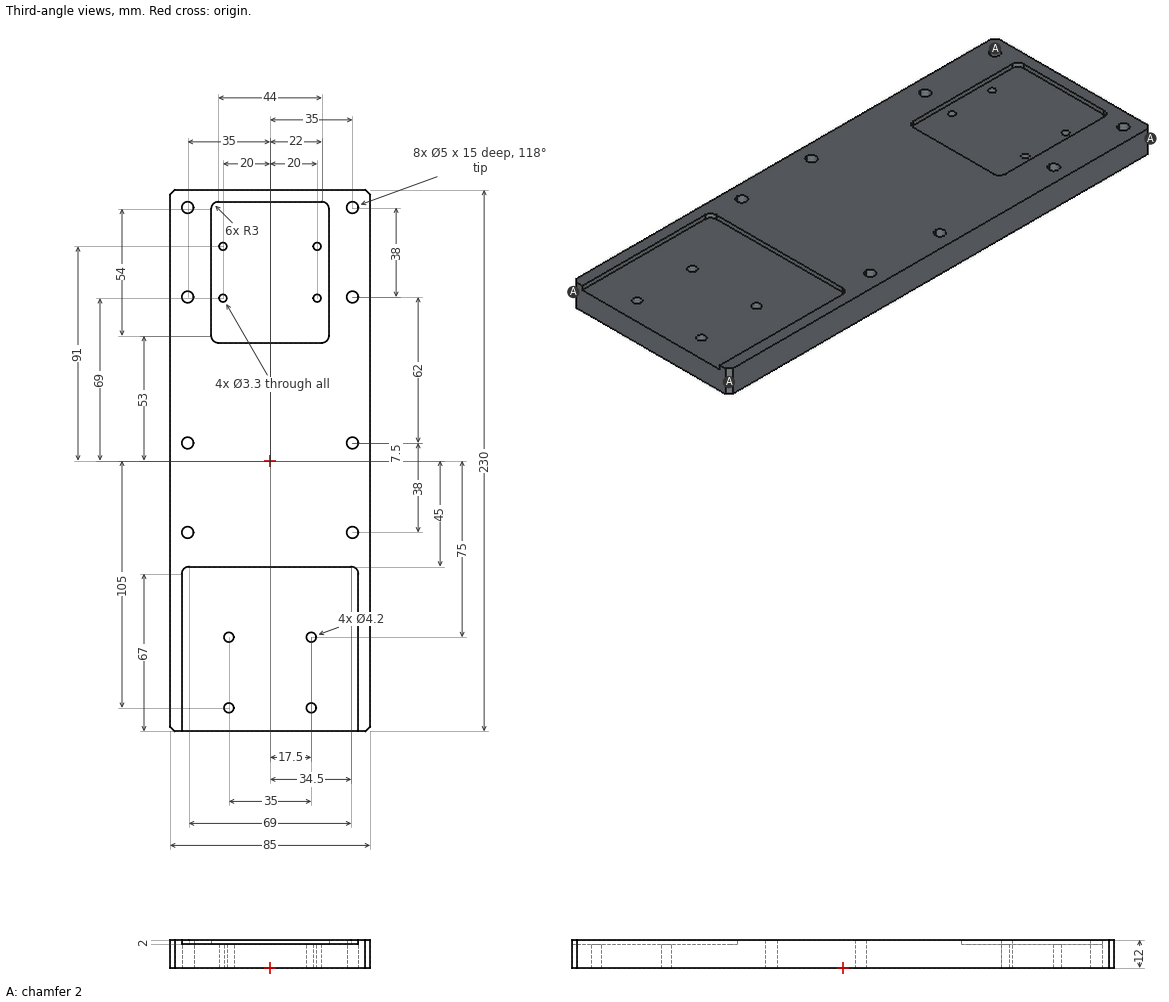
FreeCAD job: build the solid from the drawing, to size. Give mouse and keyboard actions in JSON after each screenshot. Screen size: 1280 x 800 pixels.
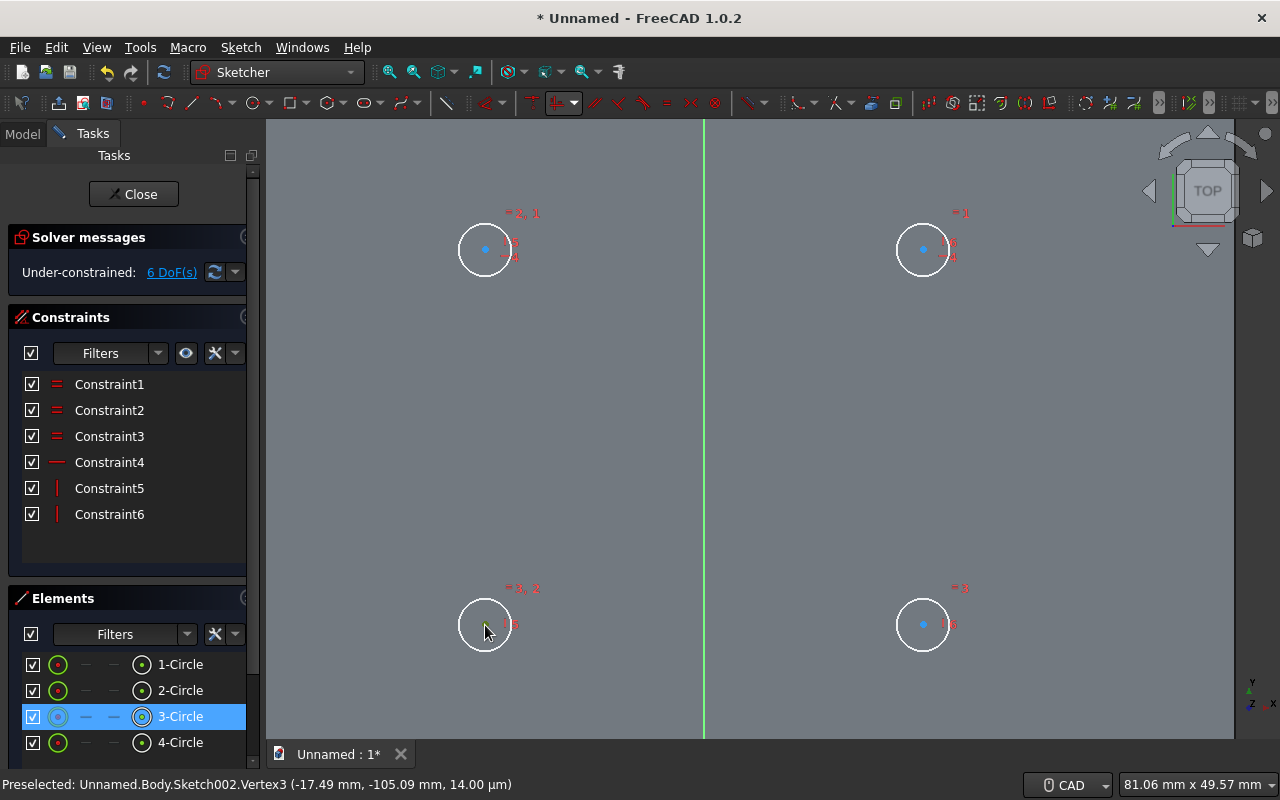
{"action": "left_click", "coordinate": [923, 625]}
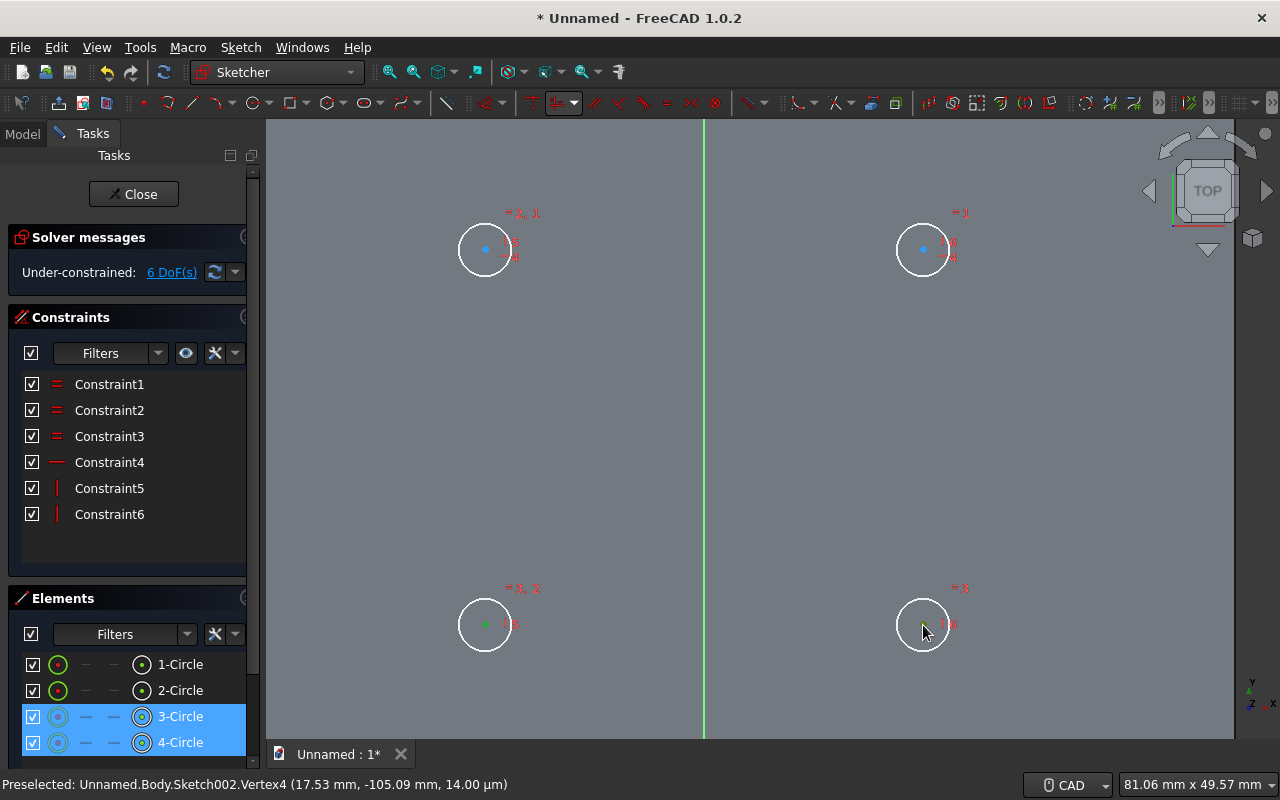
{"action": "key", "text": "h"}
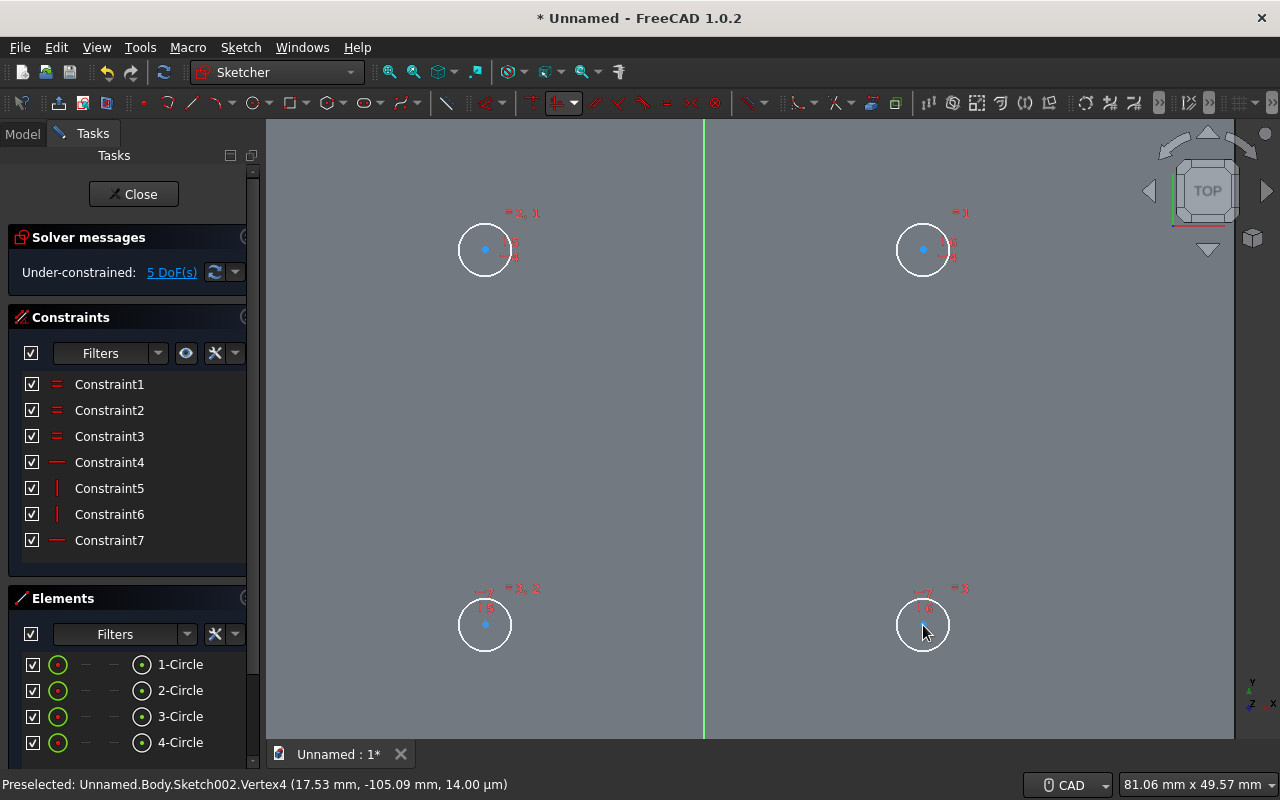
{"action": "left_click", "coordinate": [941, 231]}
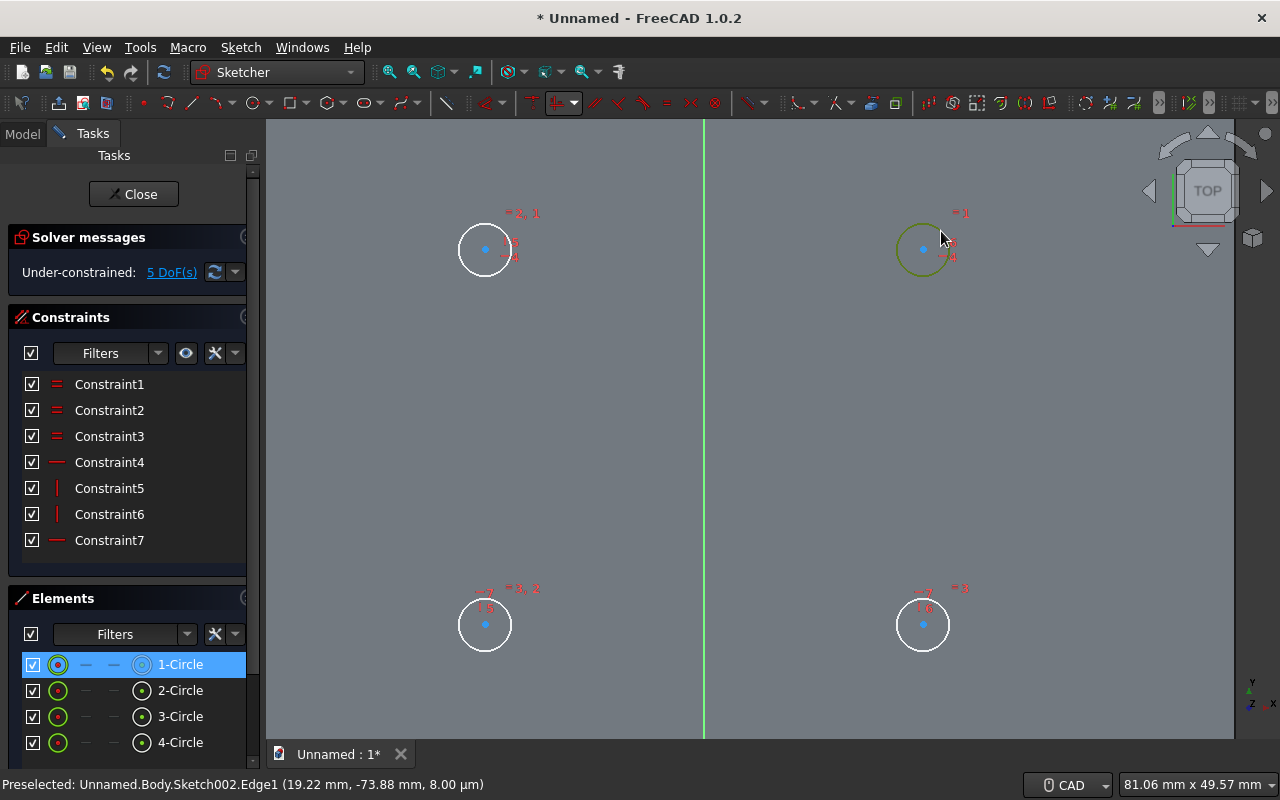
{"action": "left_click", "coordinate": [504, 104]}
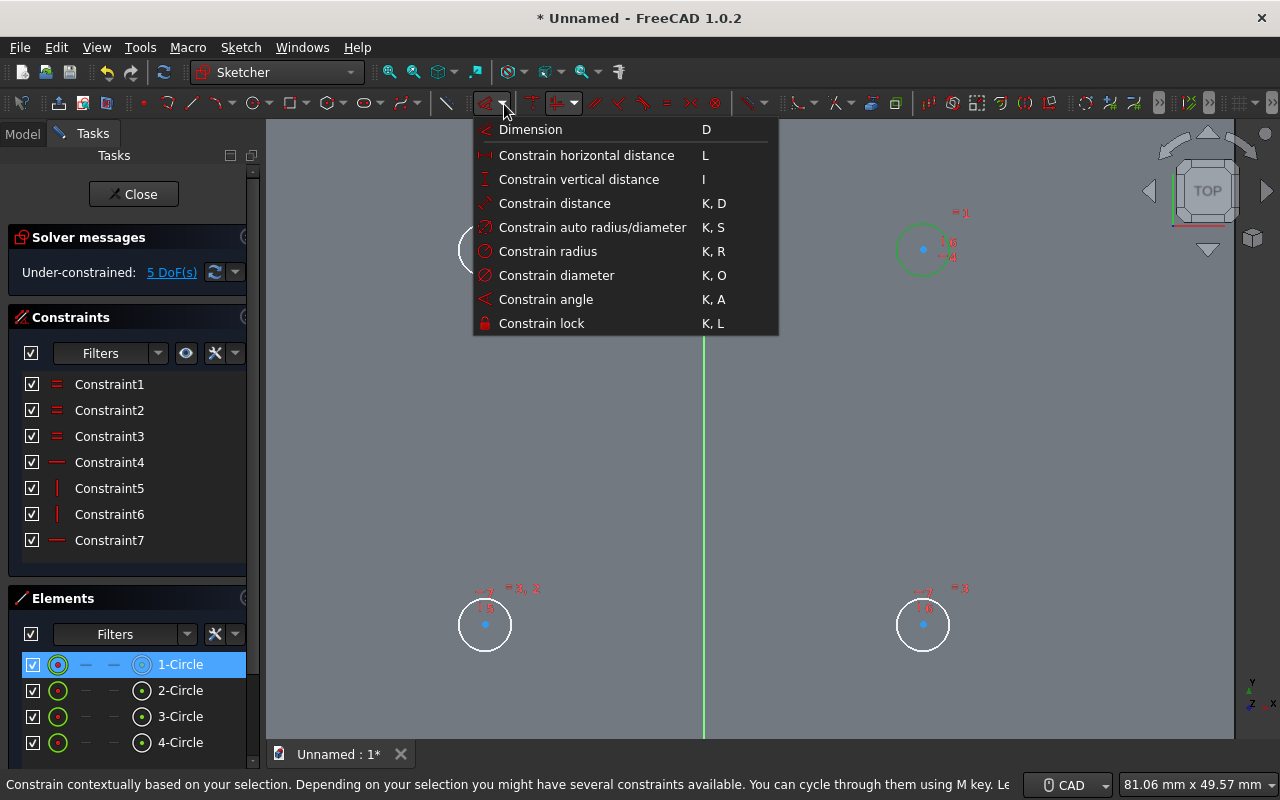
{"action": "left_click", "coordinate": [626, 275]}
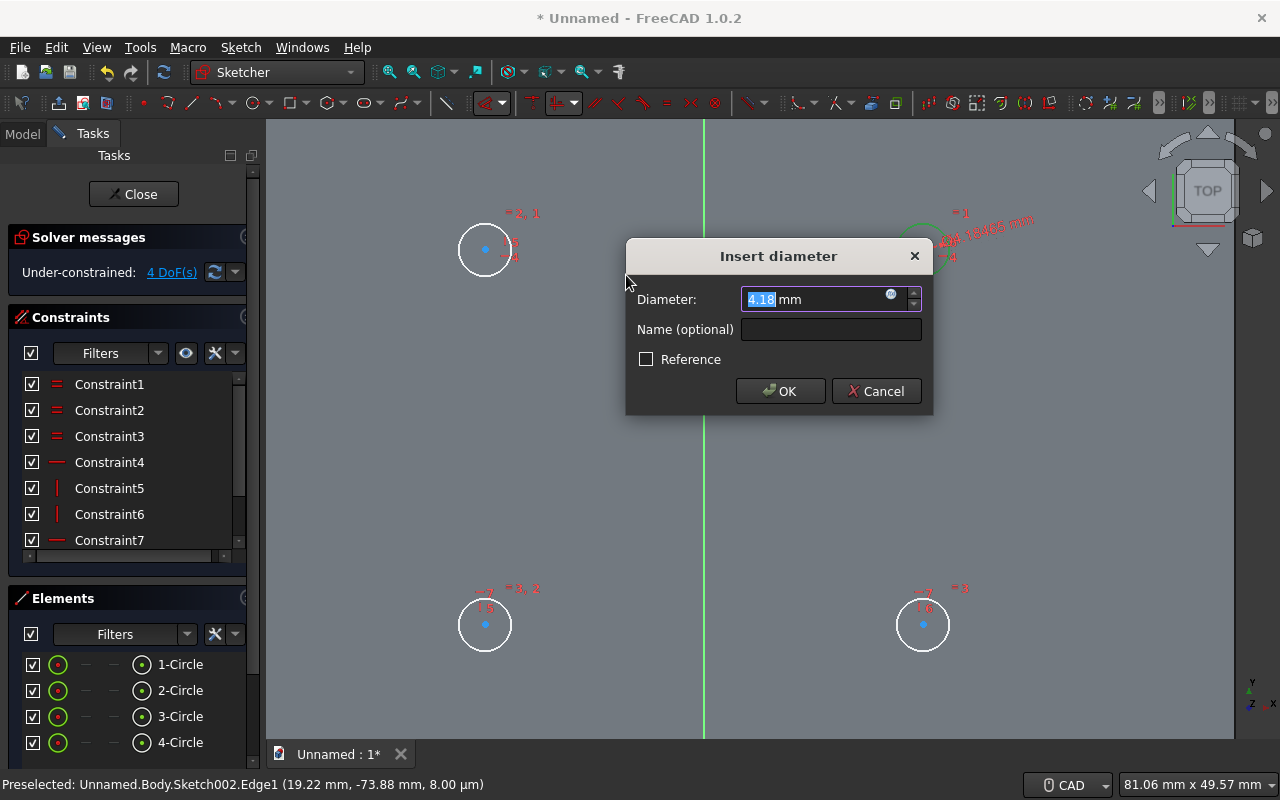
{"action": "type", "text": "4.2"}
{"action": "key", "text": "Return"}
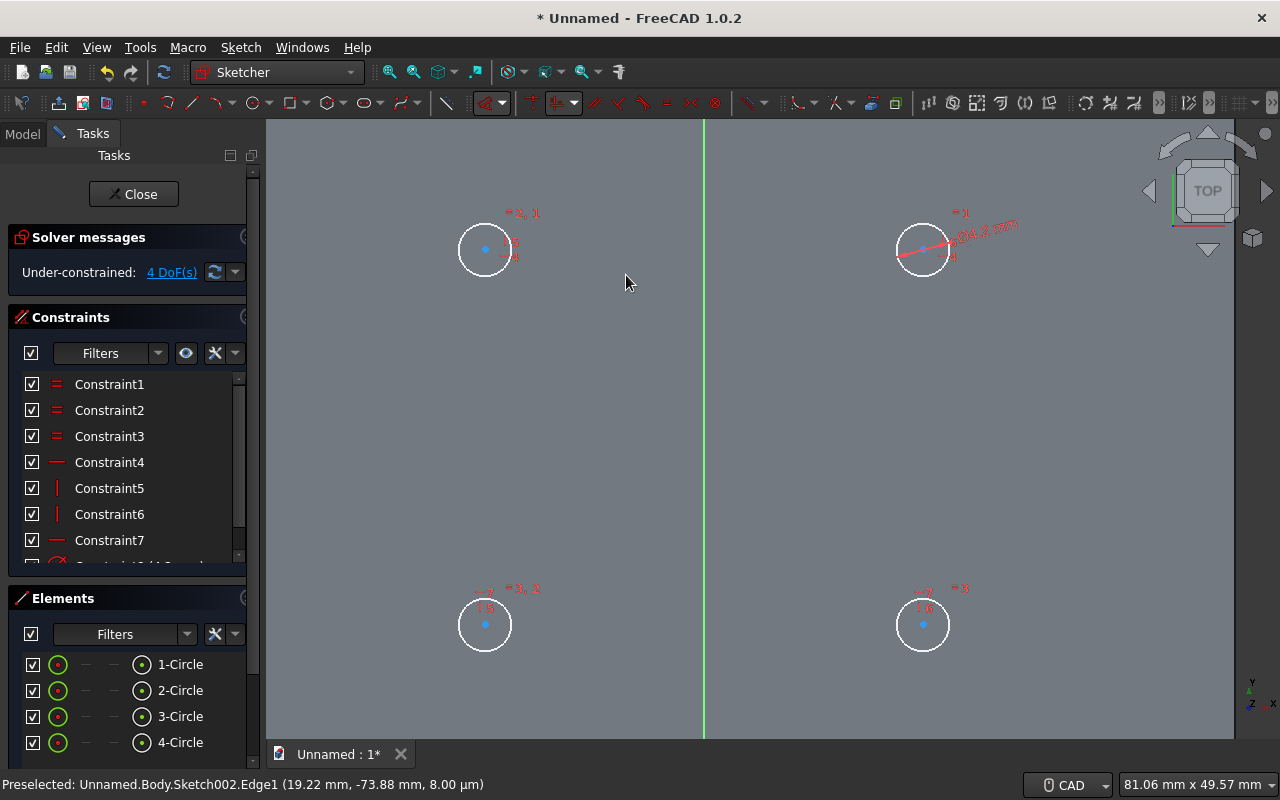
{"action": "left_click", "coordinate": [923, 250]}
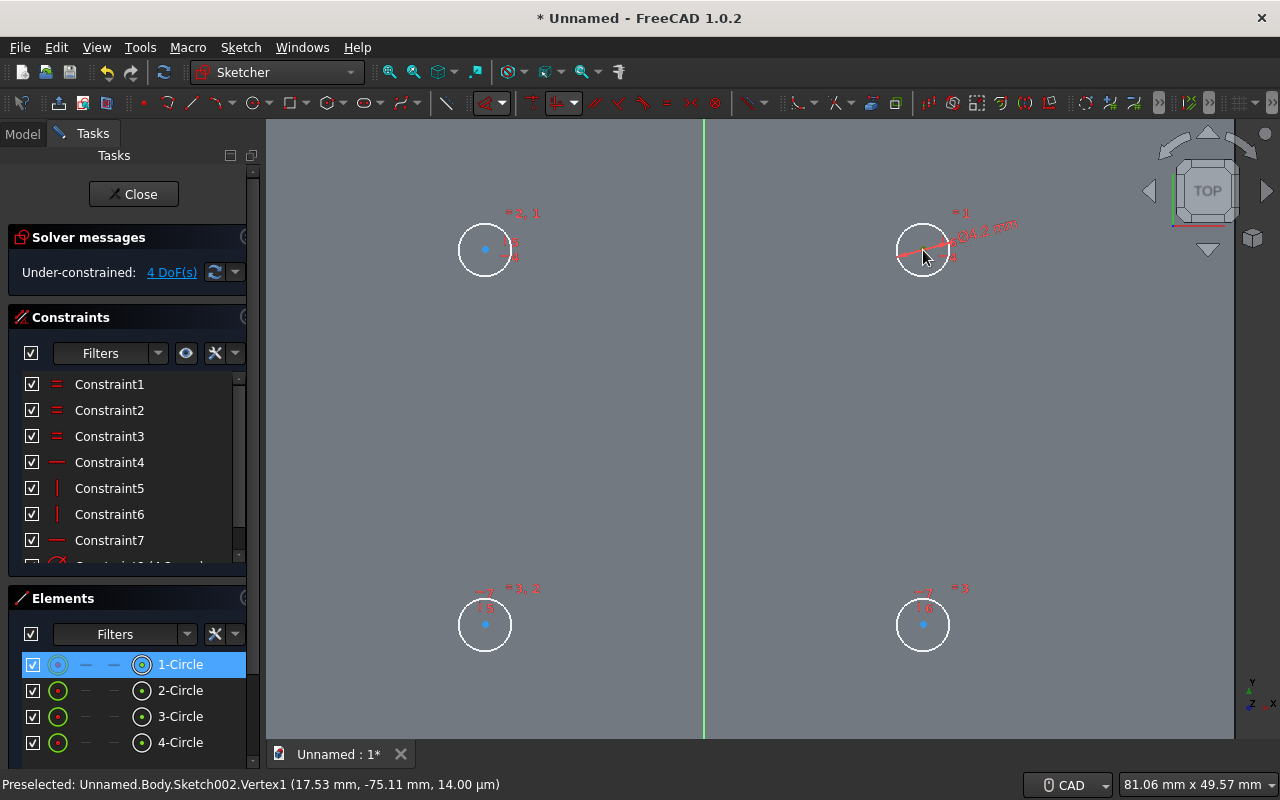
{"action": "key", "text": "i"}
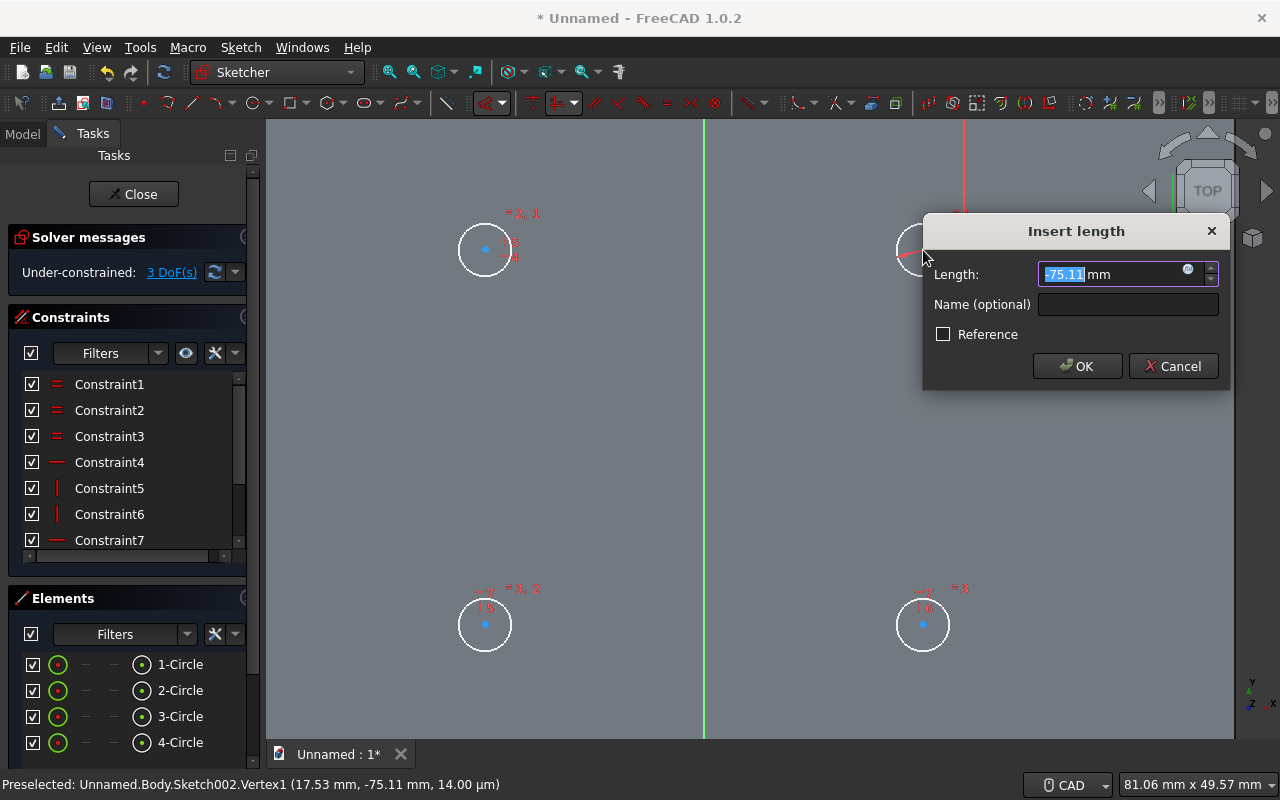
{"action": "type", "text": "-75"}
{"action": "key", "text": "Return"}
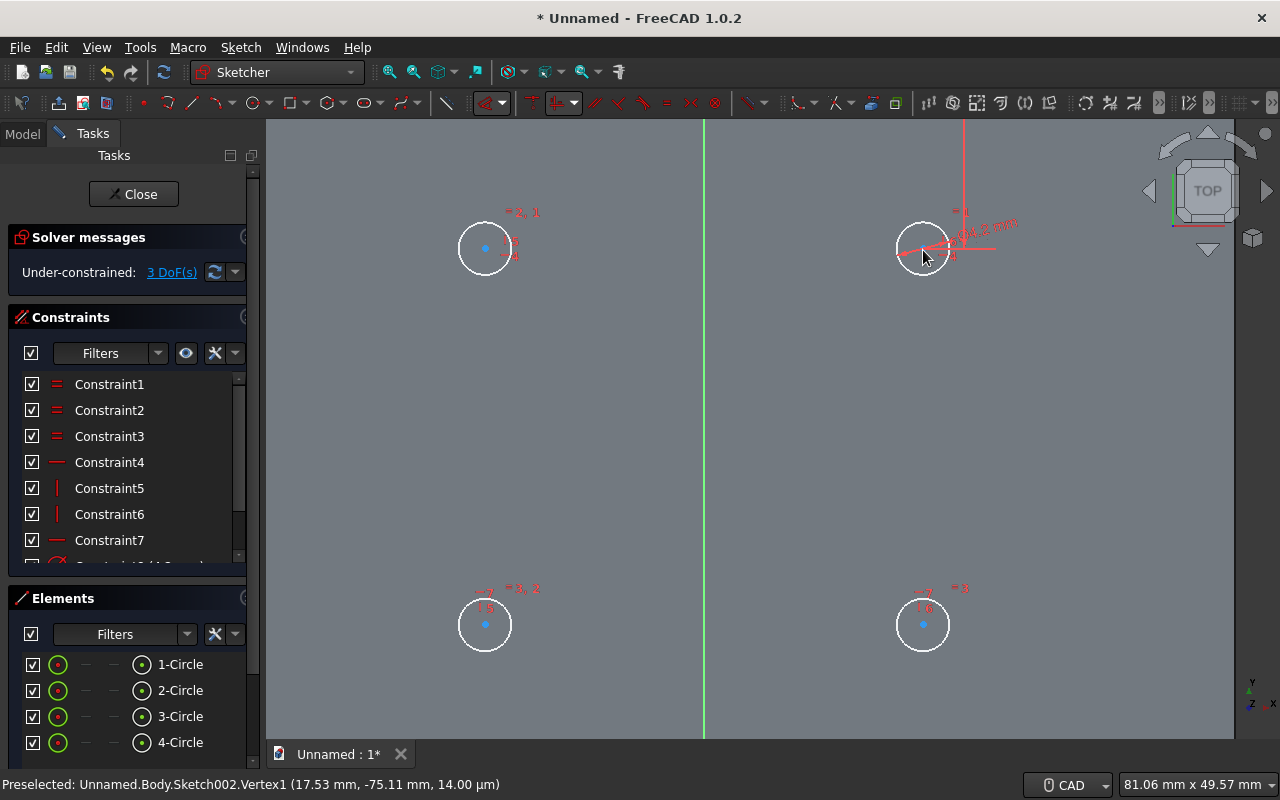
{"action": "left_click", "coordinate": [485, 625]}